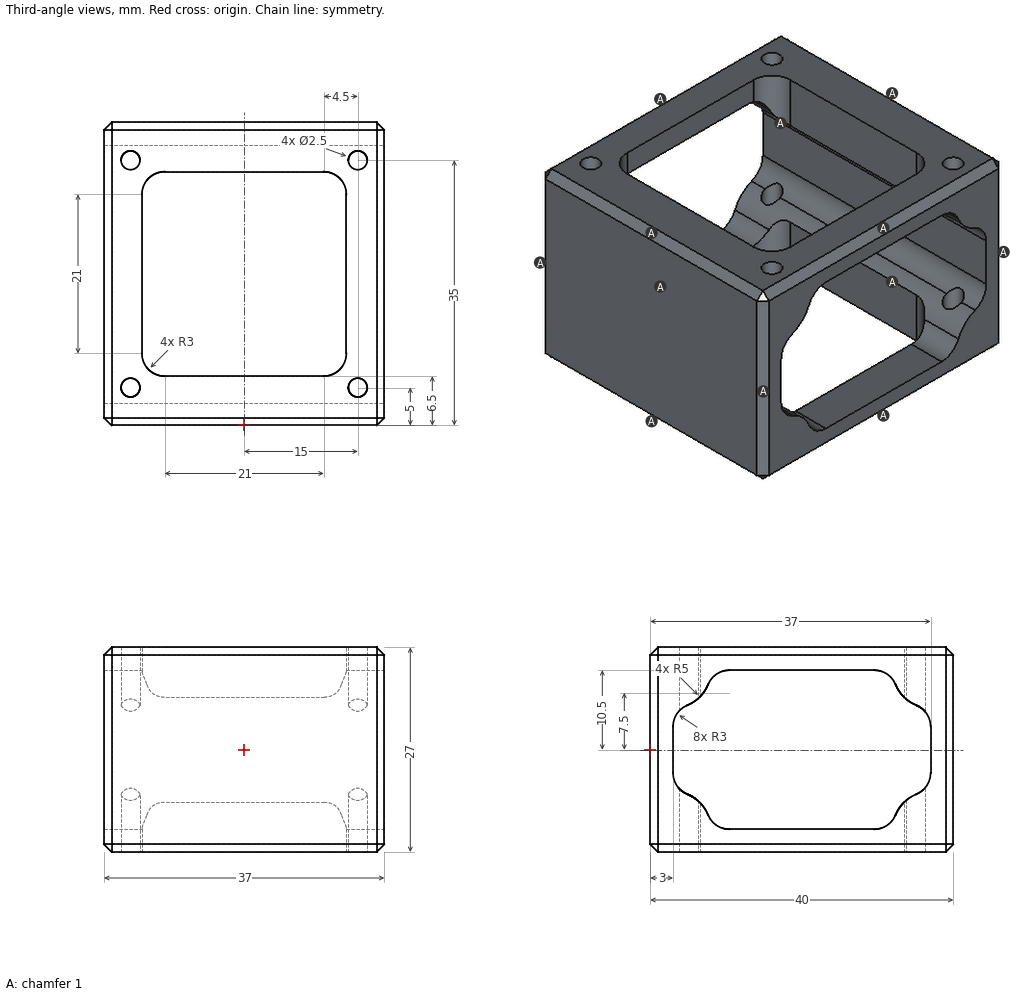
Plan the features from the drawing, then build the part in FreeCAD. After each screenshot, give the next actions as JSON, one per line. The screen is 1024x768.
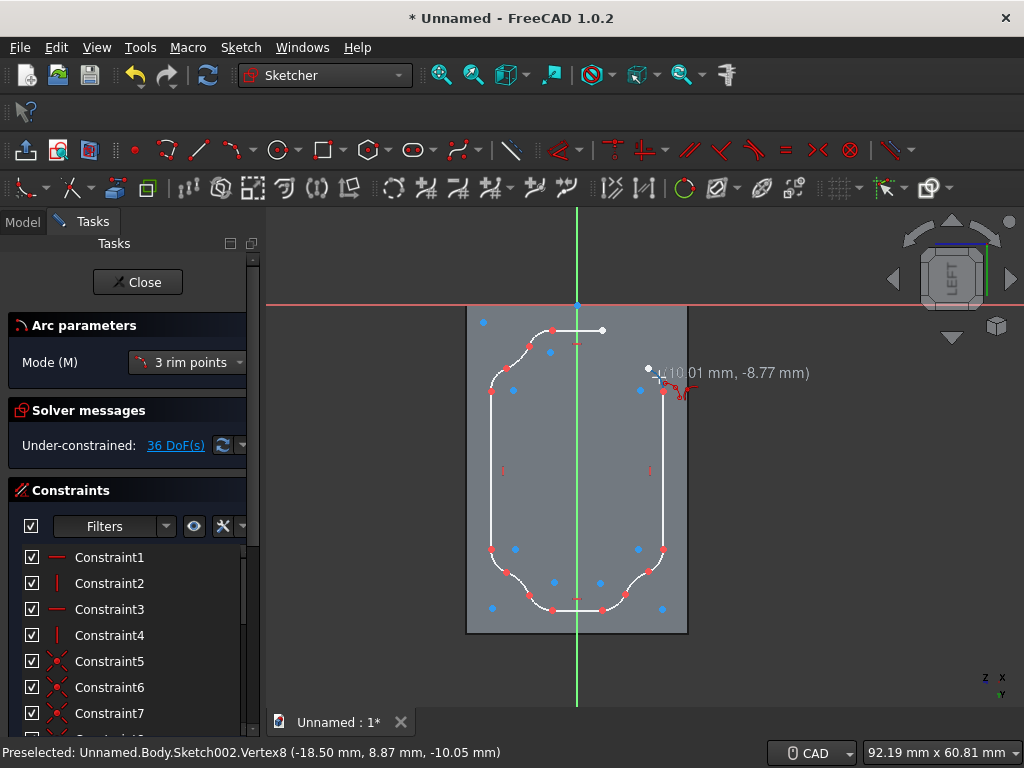
{"action": "left_click", "coordinate": [648, 369]}
{"action": "left_click", "coordinate": [625, 345]}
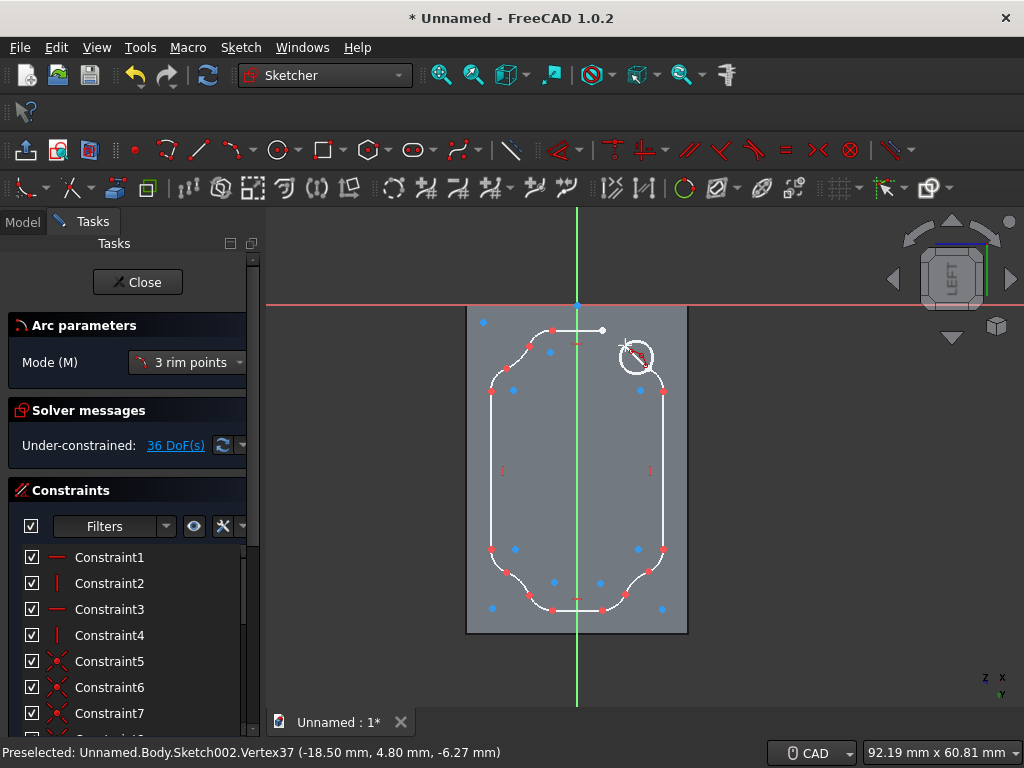
{"action": "scroll", "coordinate": [634, 359], "scroll_direction": "up", "scroll_amount": 8}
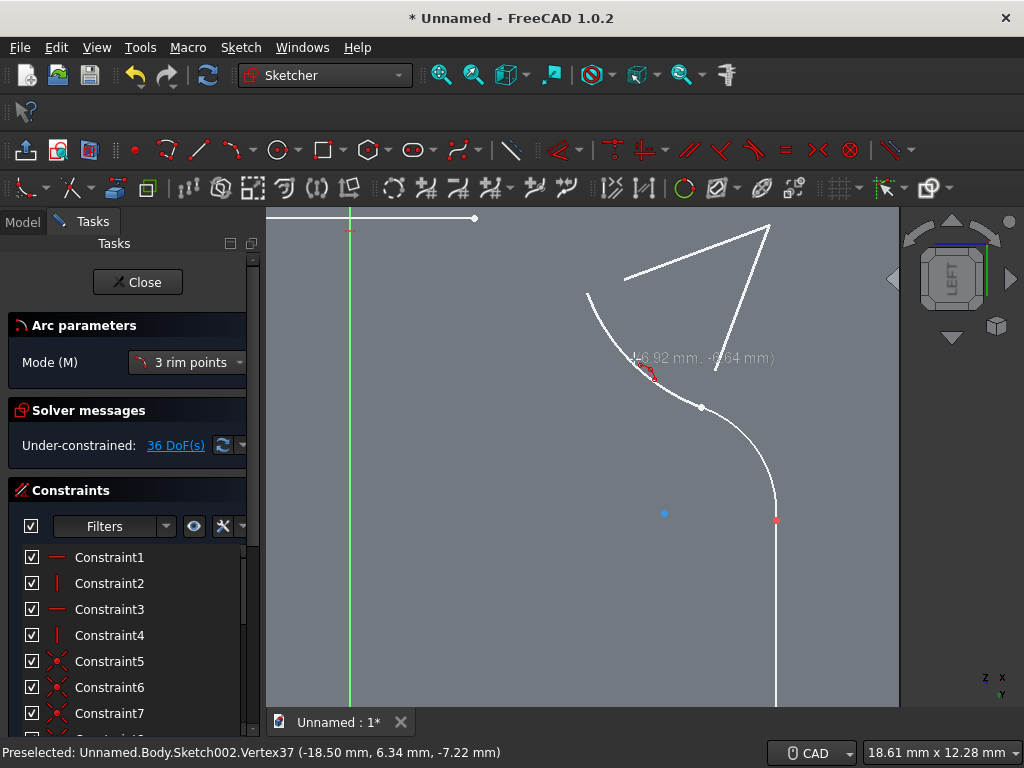
{"action": "left_click", "coordinate": [634, 358]}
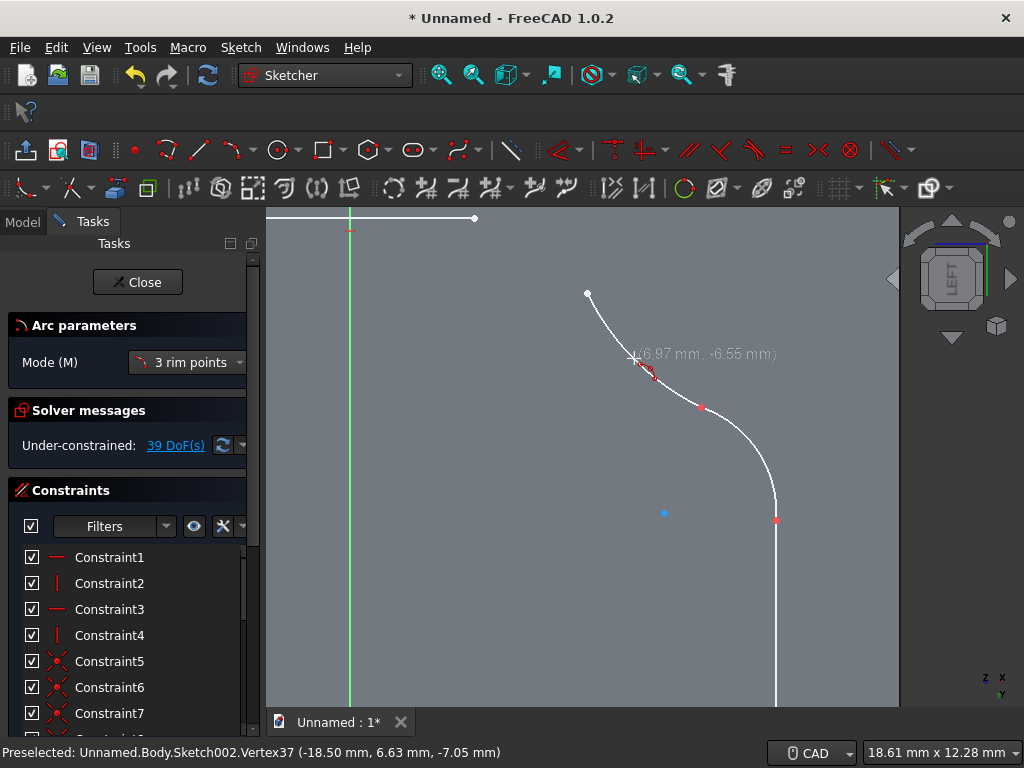
{"action": "scroll", "coordinate": [634, 359], "scroll_direction": "down", "scroll_amount": 8}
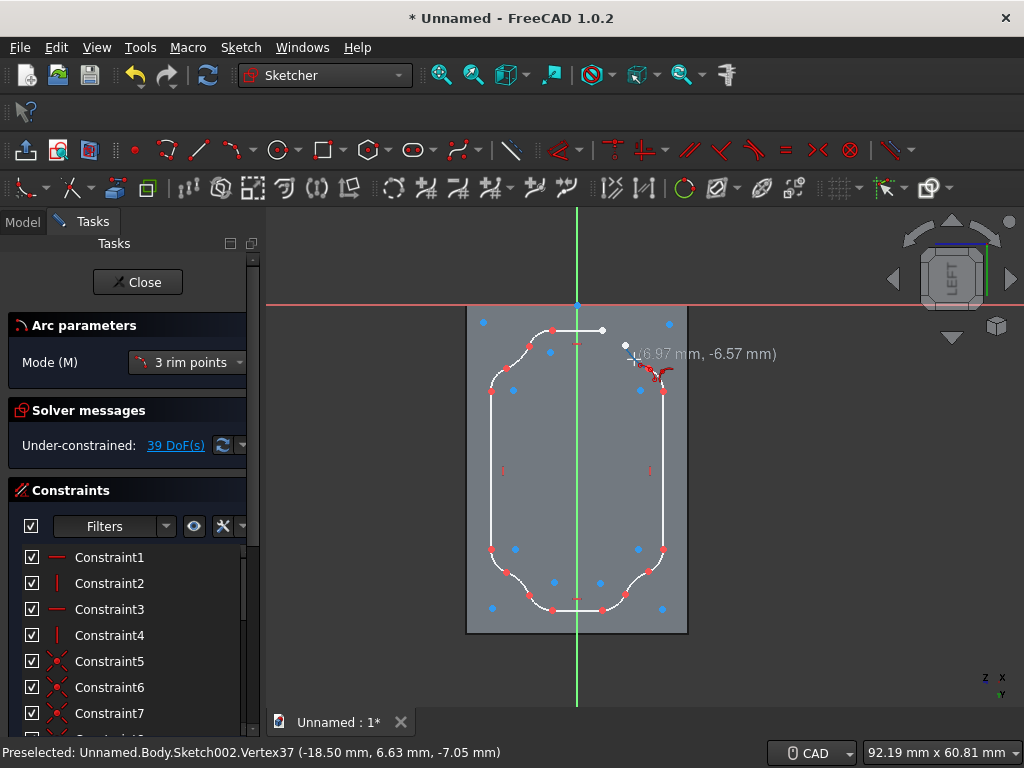
{"action": "left_click", "coordinate": [625, 346]}
{"action": "left_click", "coordinate": [602, 331]}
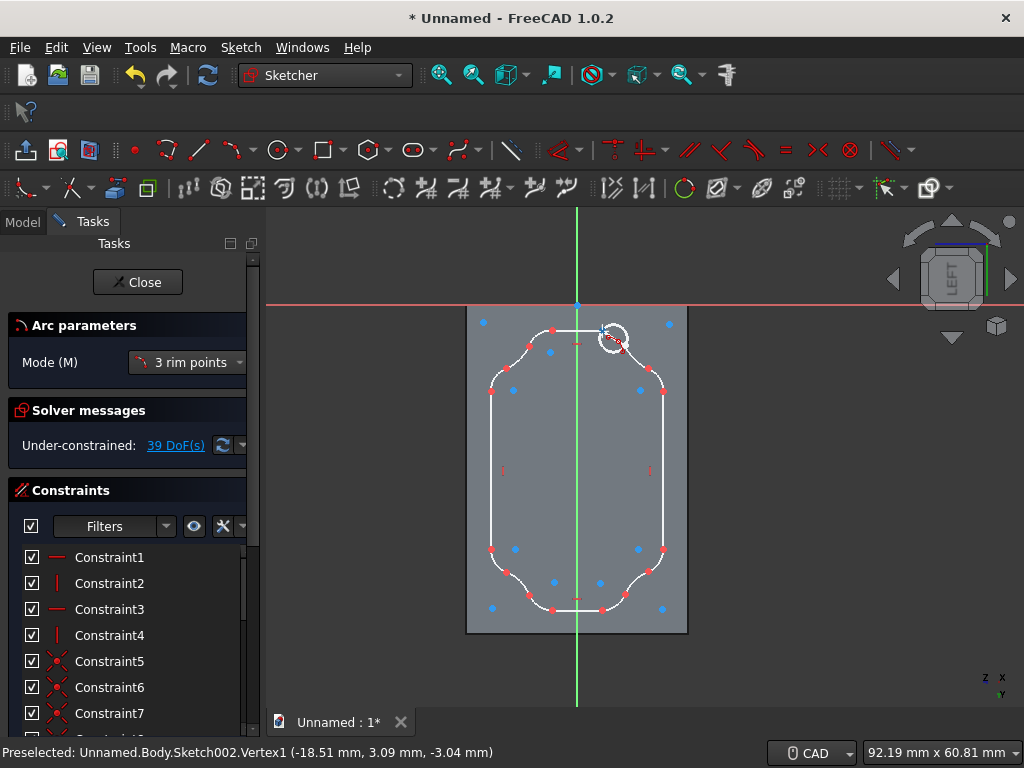
{"action": "scroll", "coordinate": [616, 334], "scroll_direction": "up", "scroll_amount": 7}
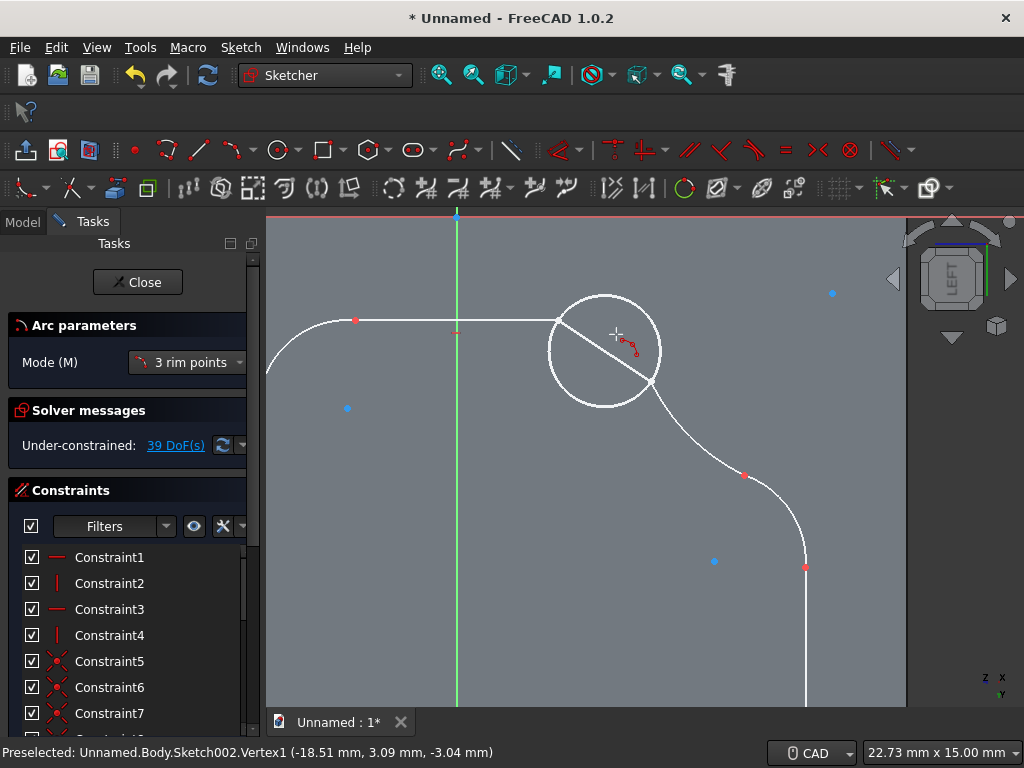
{"action": "left_click", "coordinate": [616, 334]}
{"action": "key", "text": "Escape"}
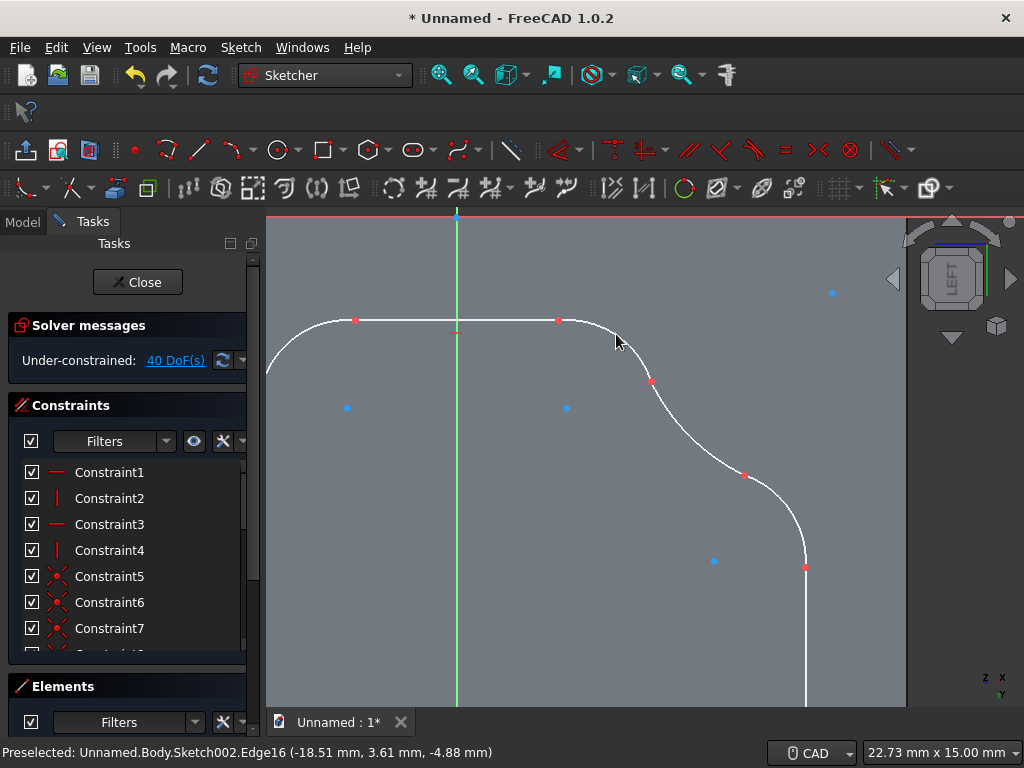
{"action": "scroll", "coordinate": [616, 334], "scroll_direction": "down", "scroll_amount": 7}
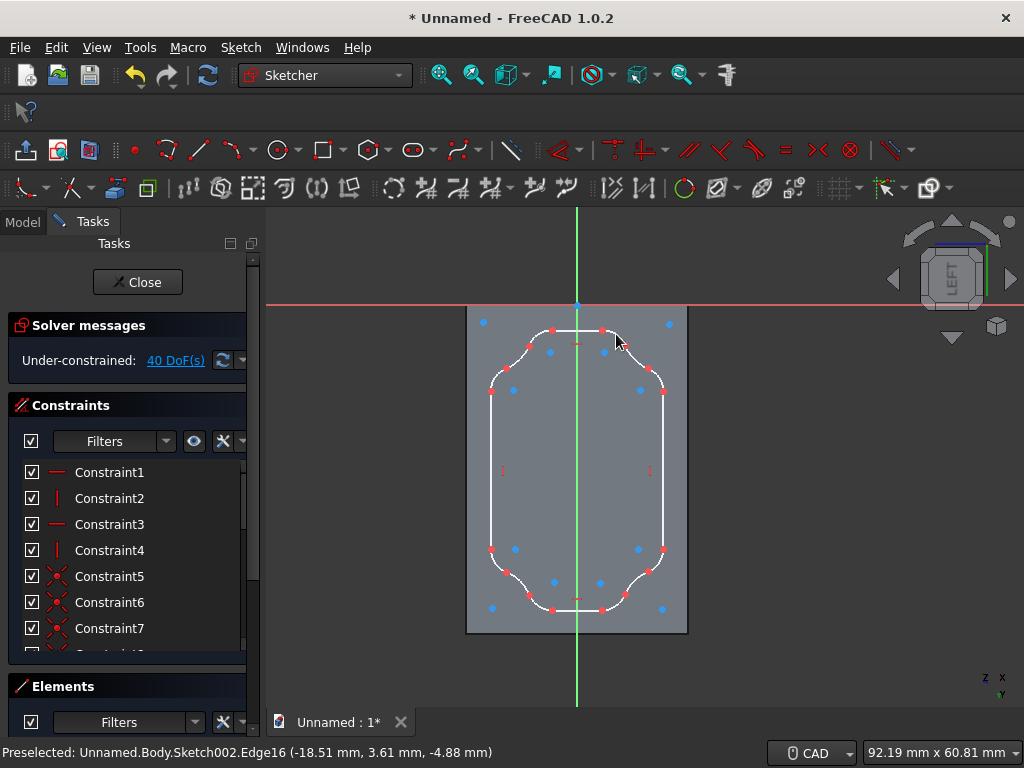
{"action": "scroll", "coordinate": [587, 331], "scroll_direction": "up", "scroll_amount": 2}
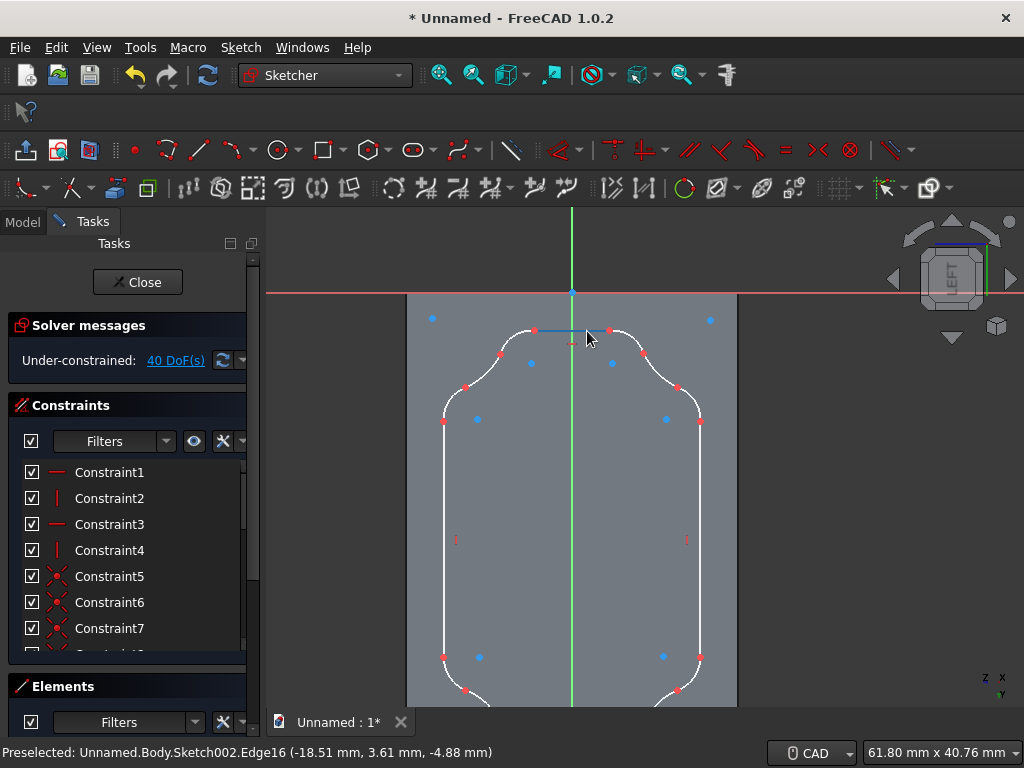
{"action": "left_click", "coordinate": [587, 331]}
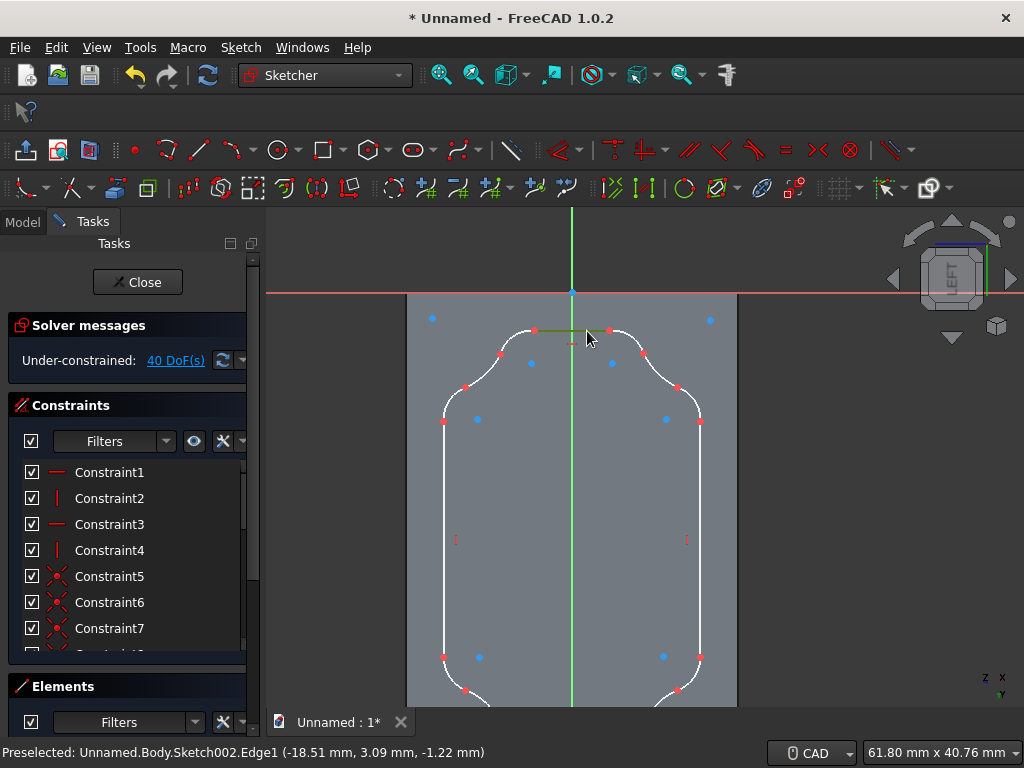
{"action": "left_click", "coordinate": [521, 332]}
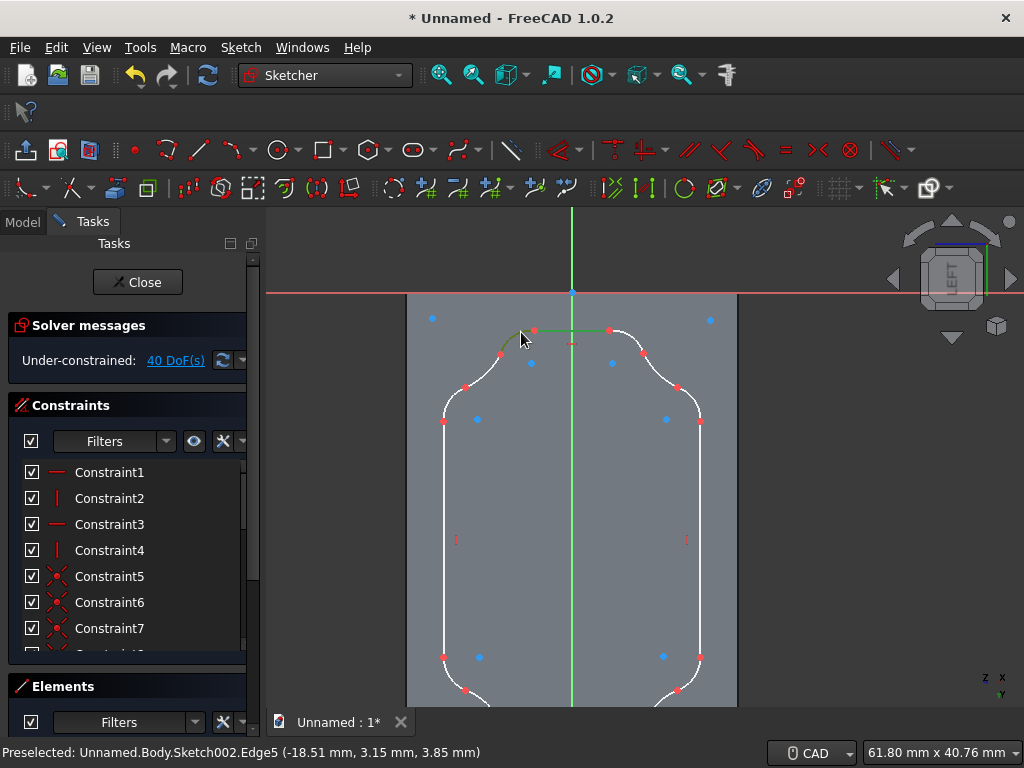
{"action": "left_click", "coordinate": [754, 150]}